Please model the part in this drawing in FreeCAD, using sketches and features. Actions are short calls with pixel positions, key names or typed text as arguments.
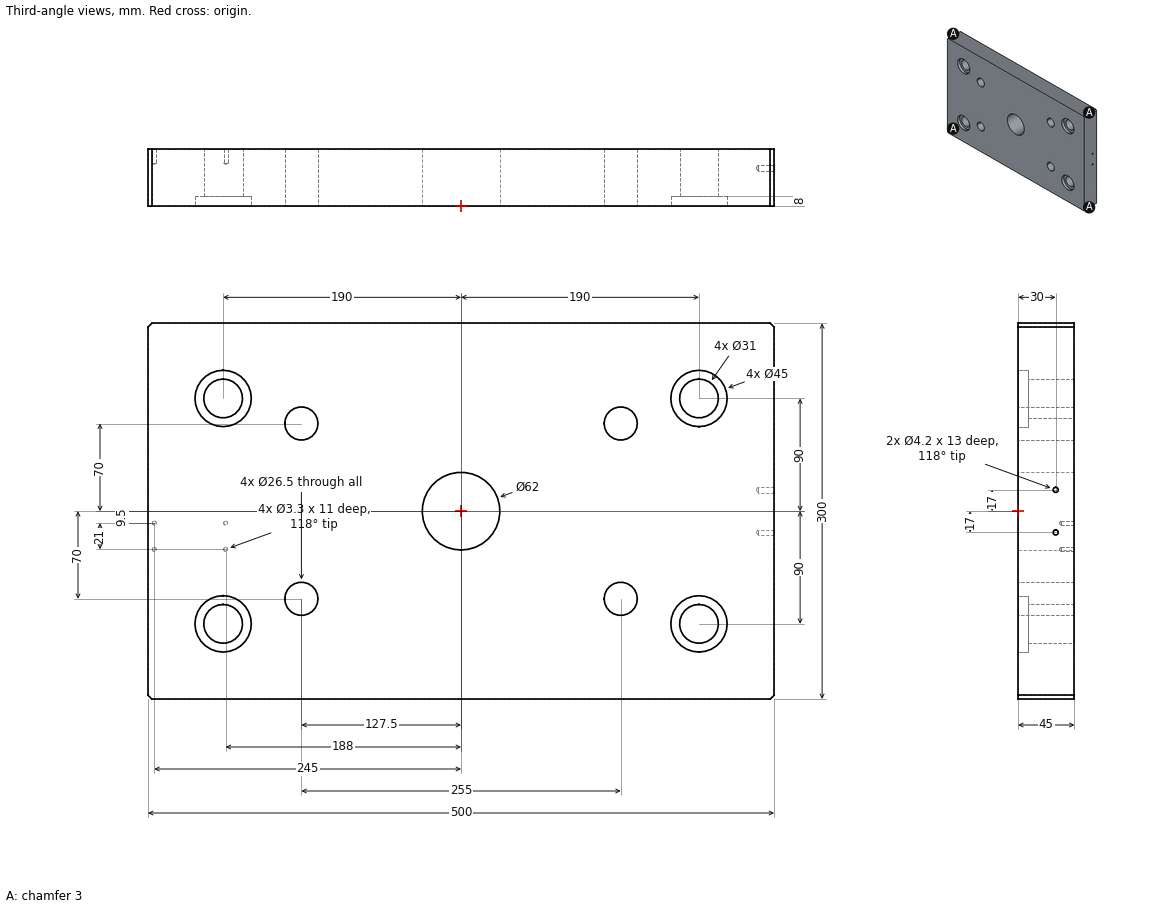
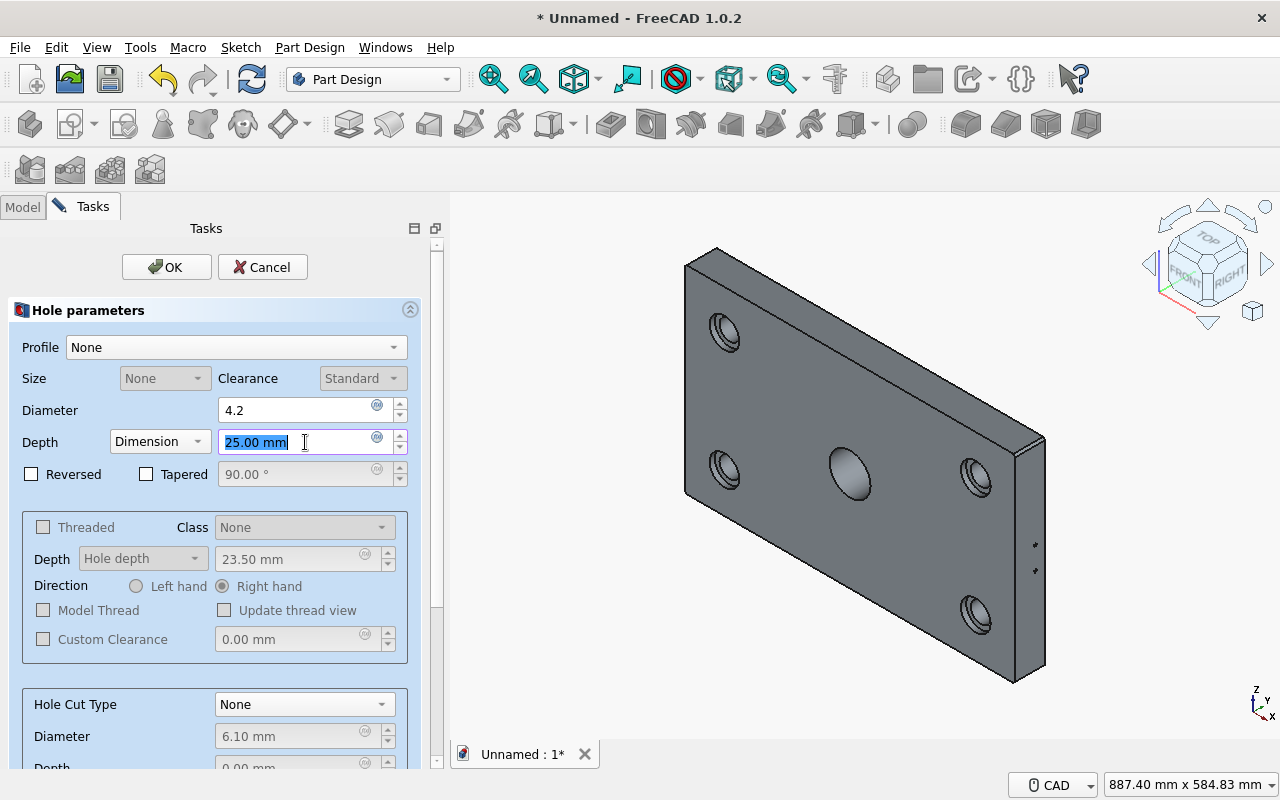
text(13)
key(Tab)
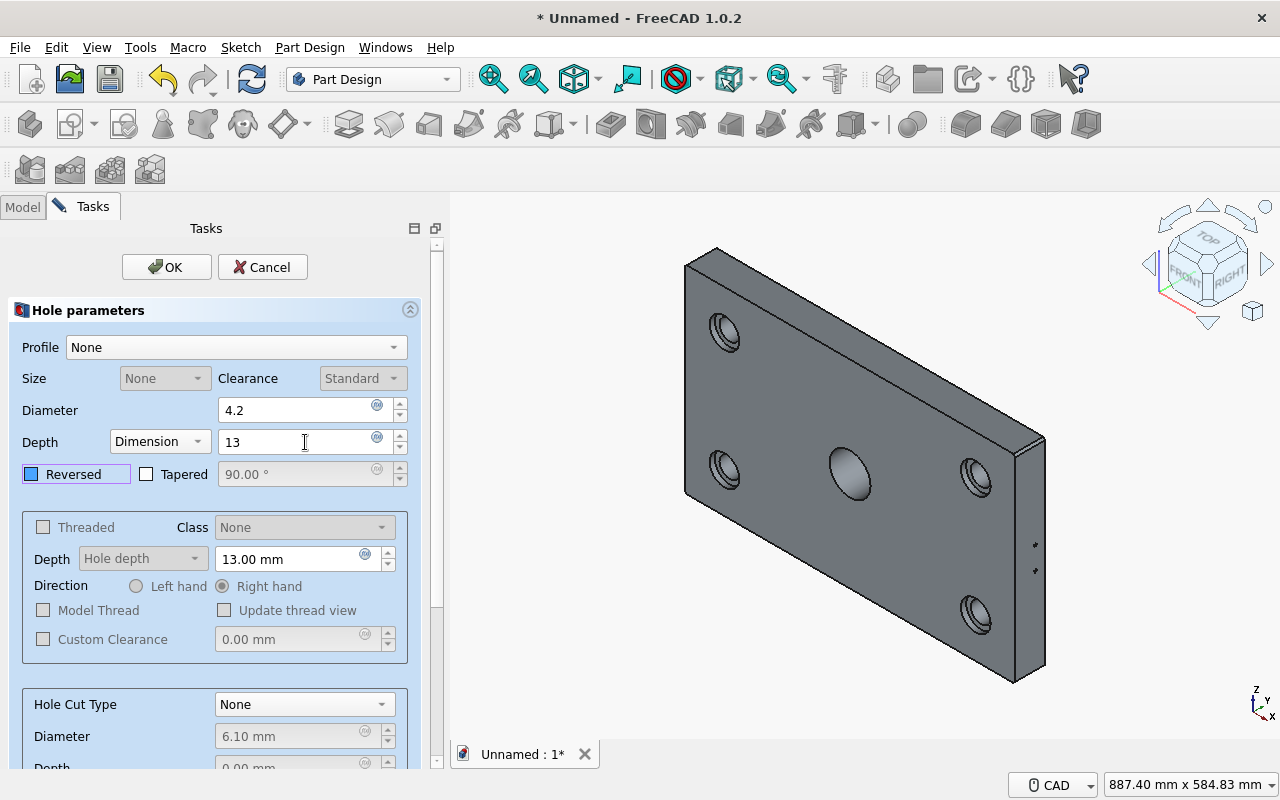
click(167, 267)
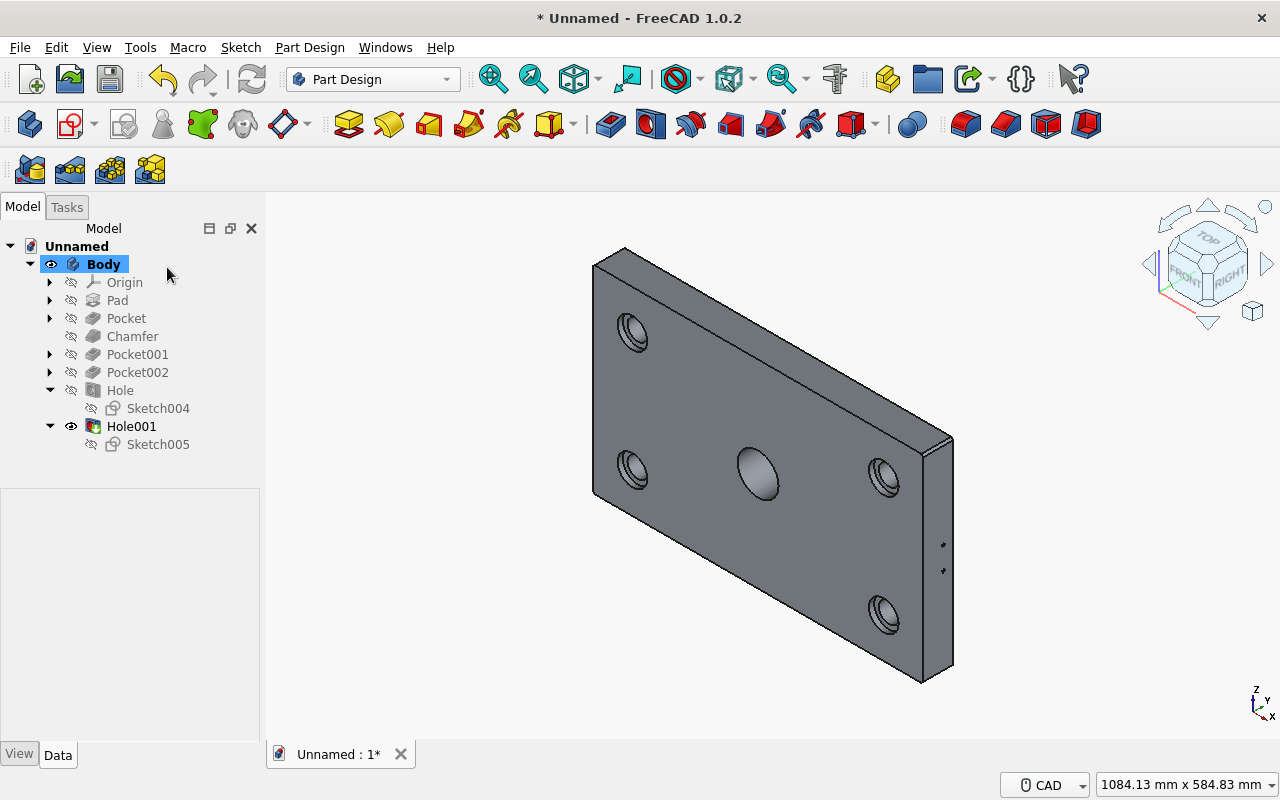
key(4)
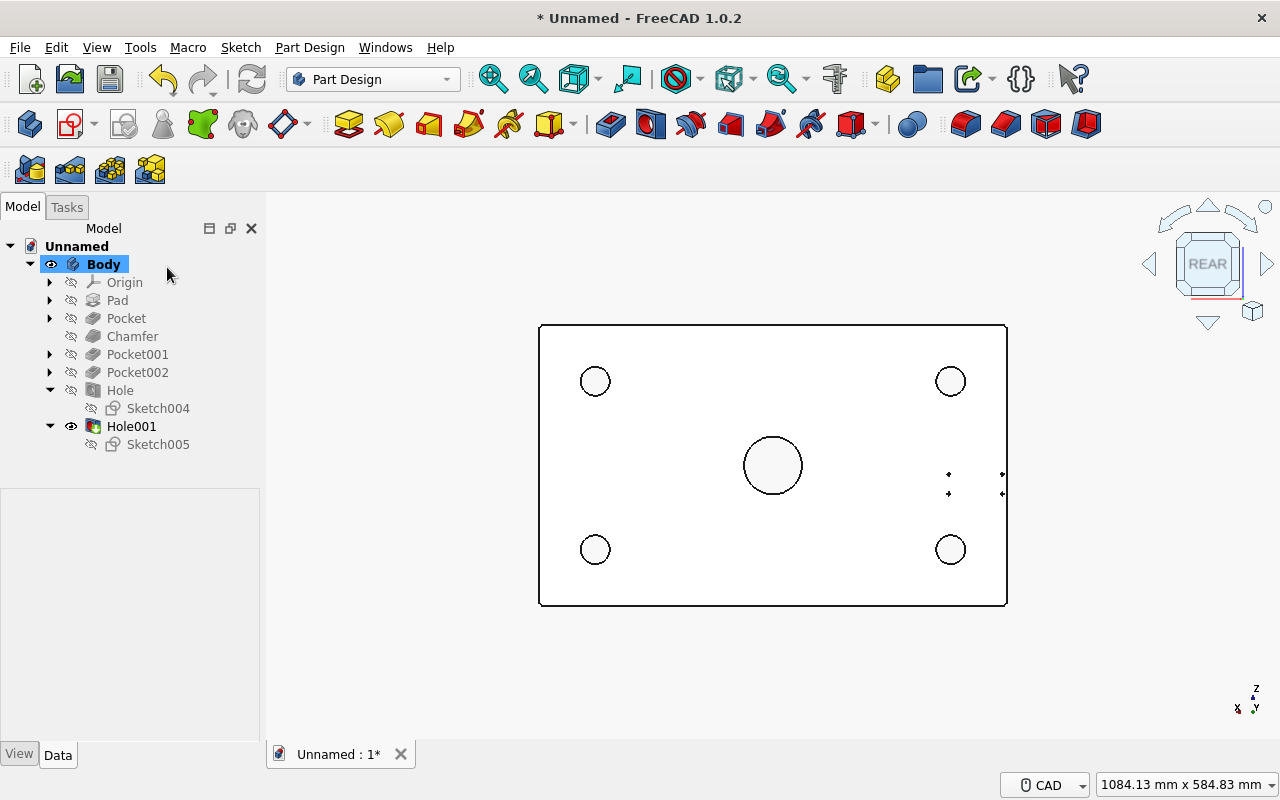
click(639, 465)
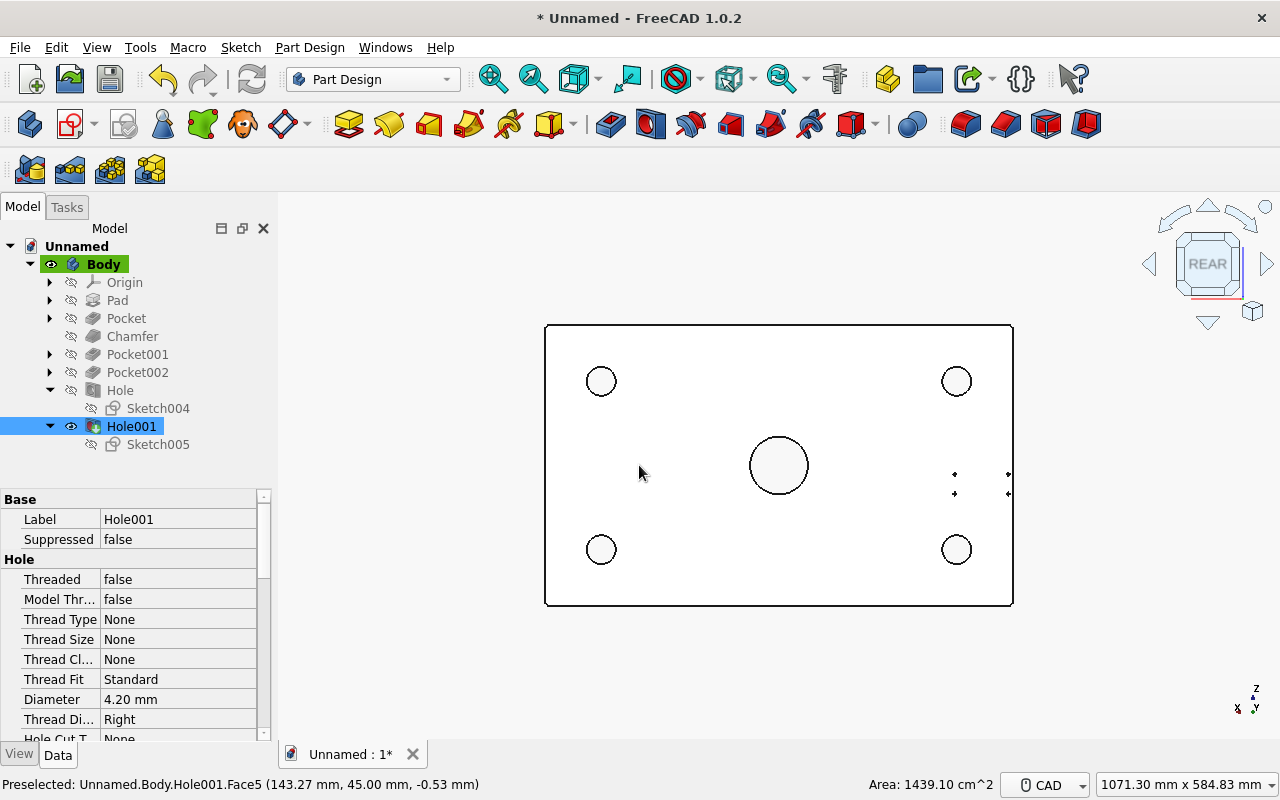
click(70, 124)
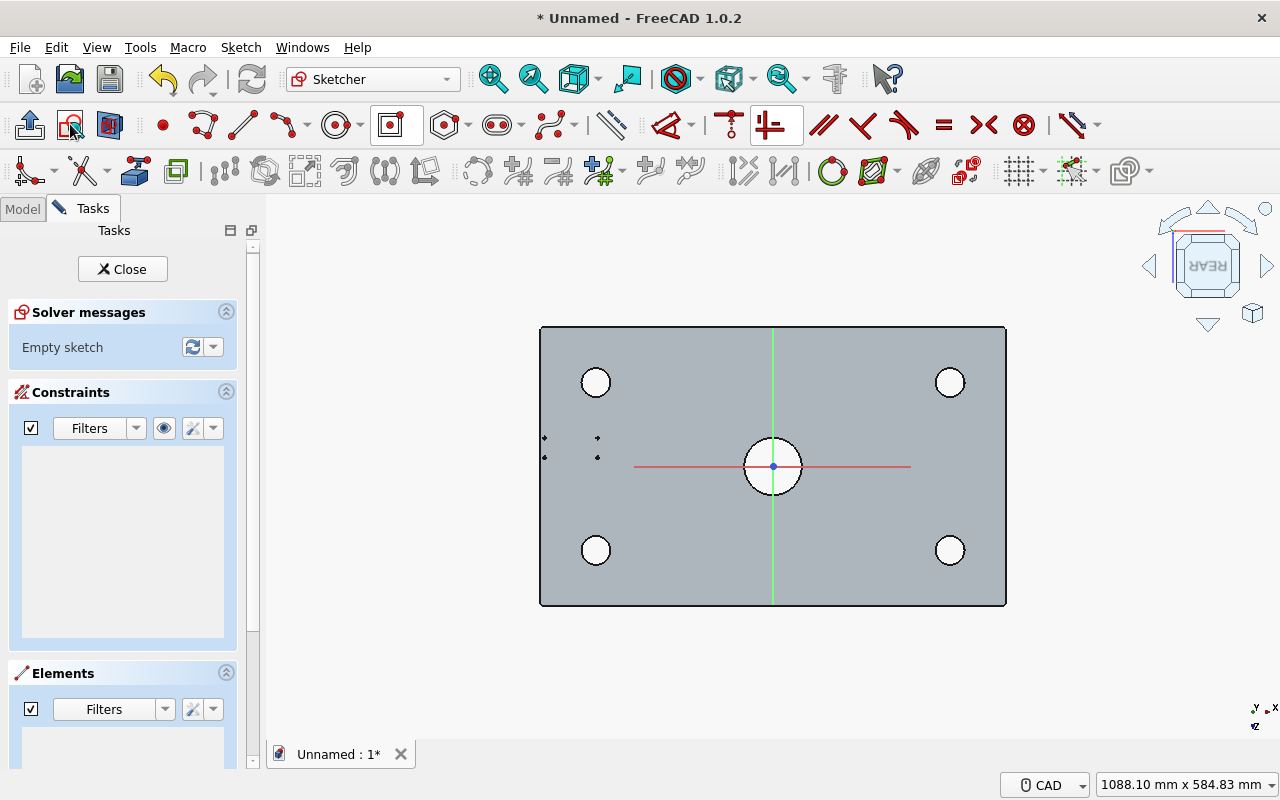
scroll(829, 466, up, 4)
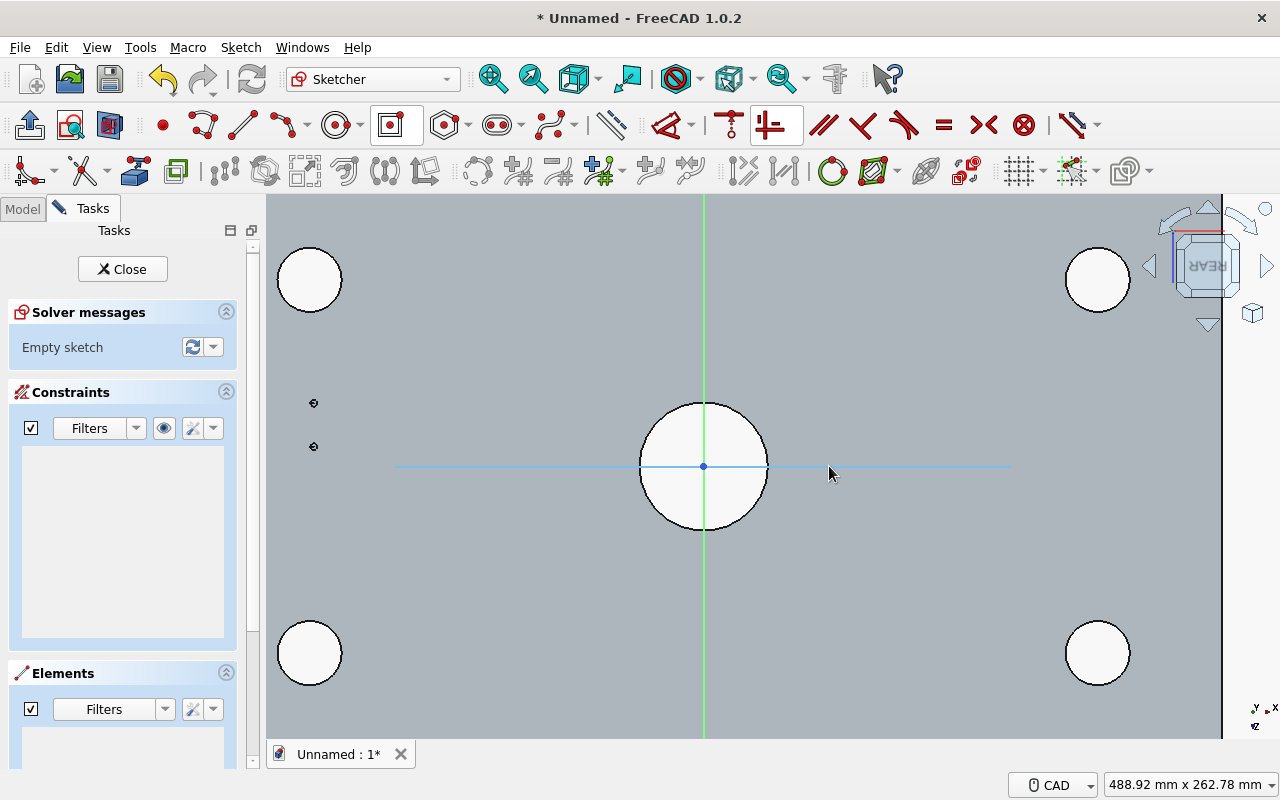
key(g)
key(c)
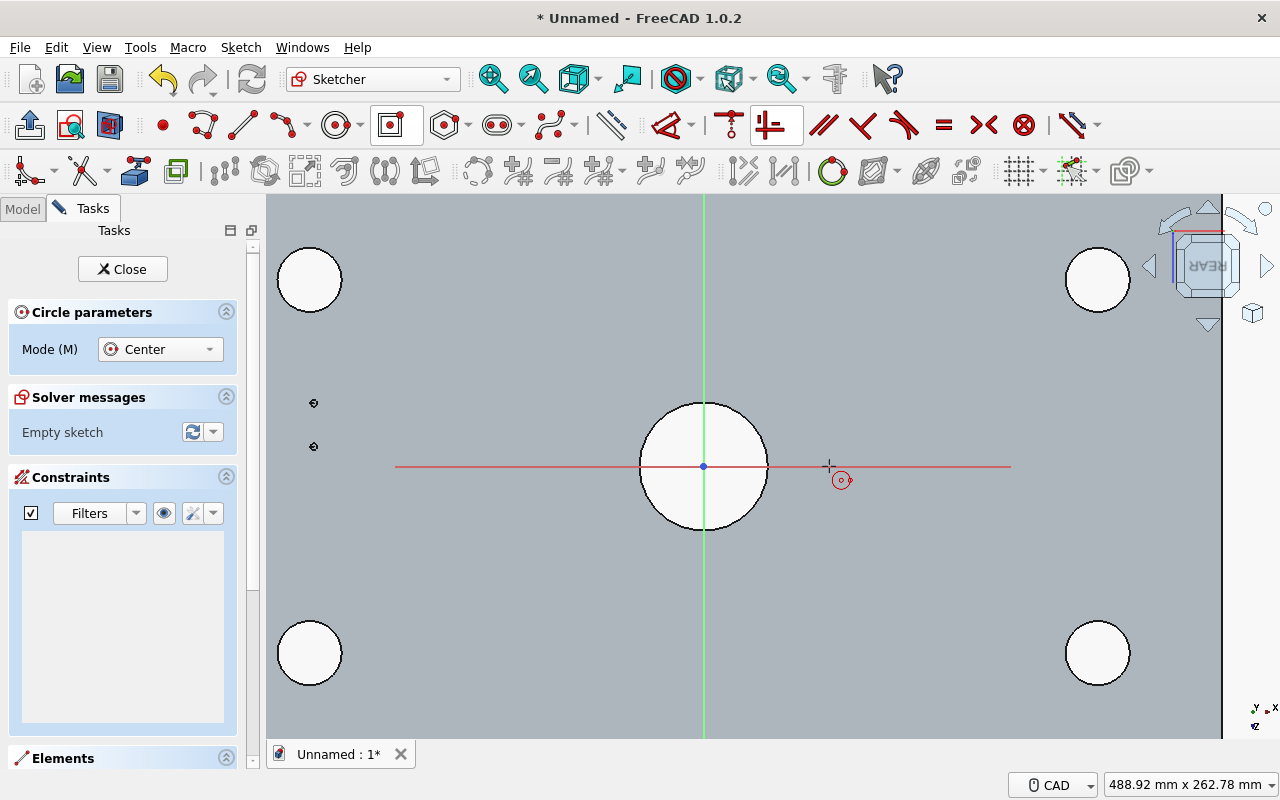
click(439, 321)
click(459, 302)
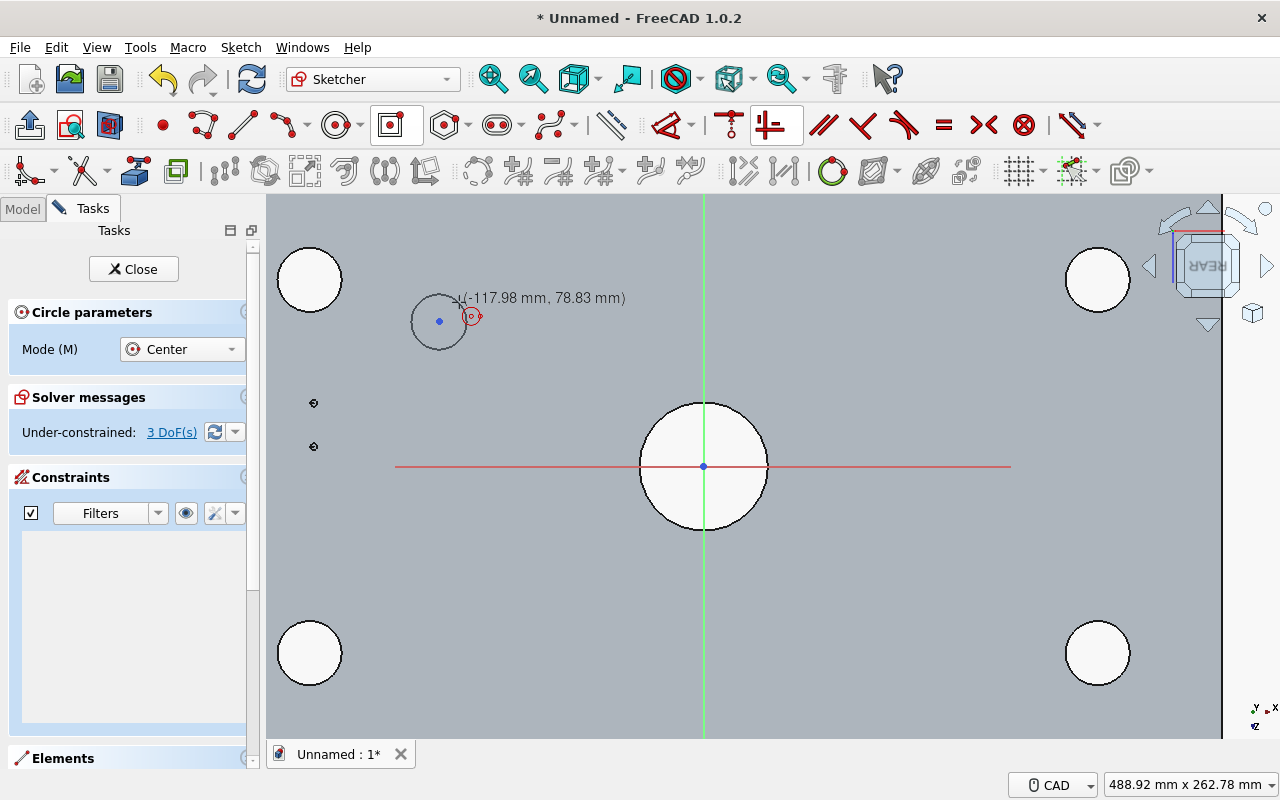
click(439, 612)
click(459, 592)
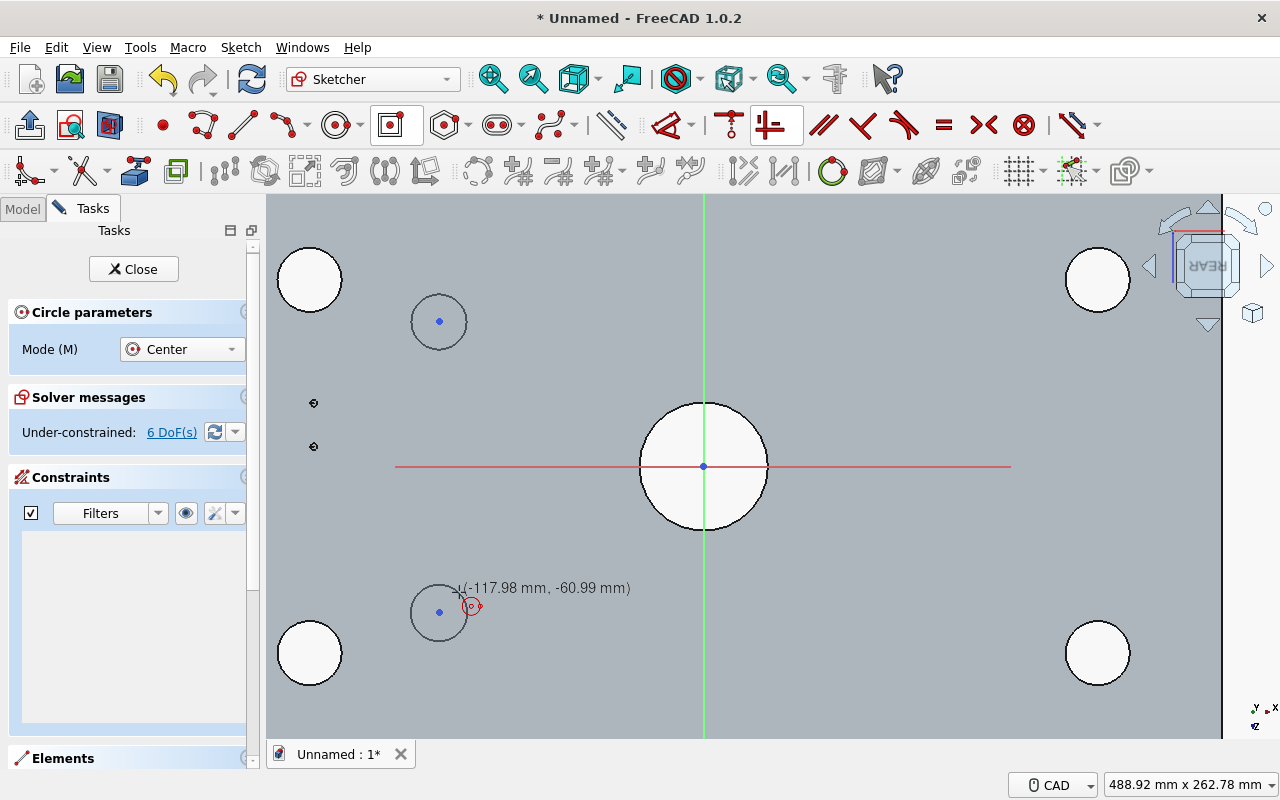
click(968, 321)
click(988, 302)